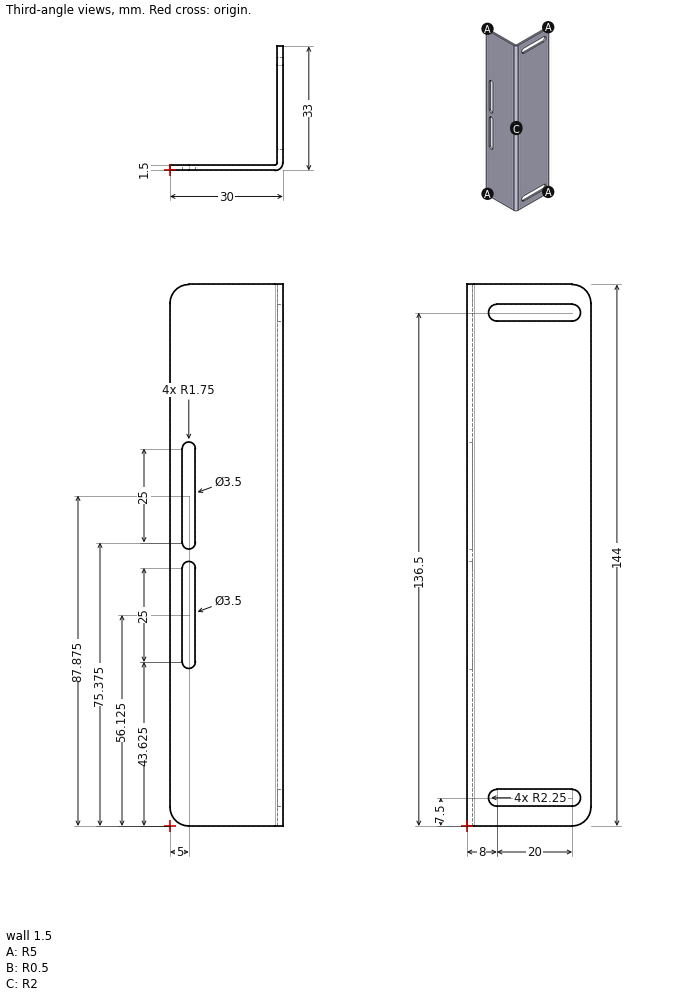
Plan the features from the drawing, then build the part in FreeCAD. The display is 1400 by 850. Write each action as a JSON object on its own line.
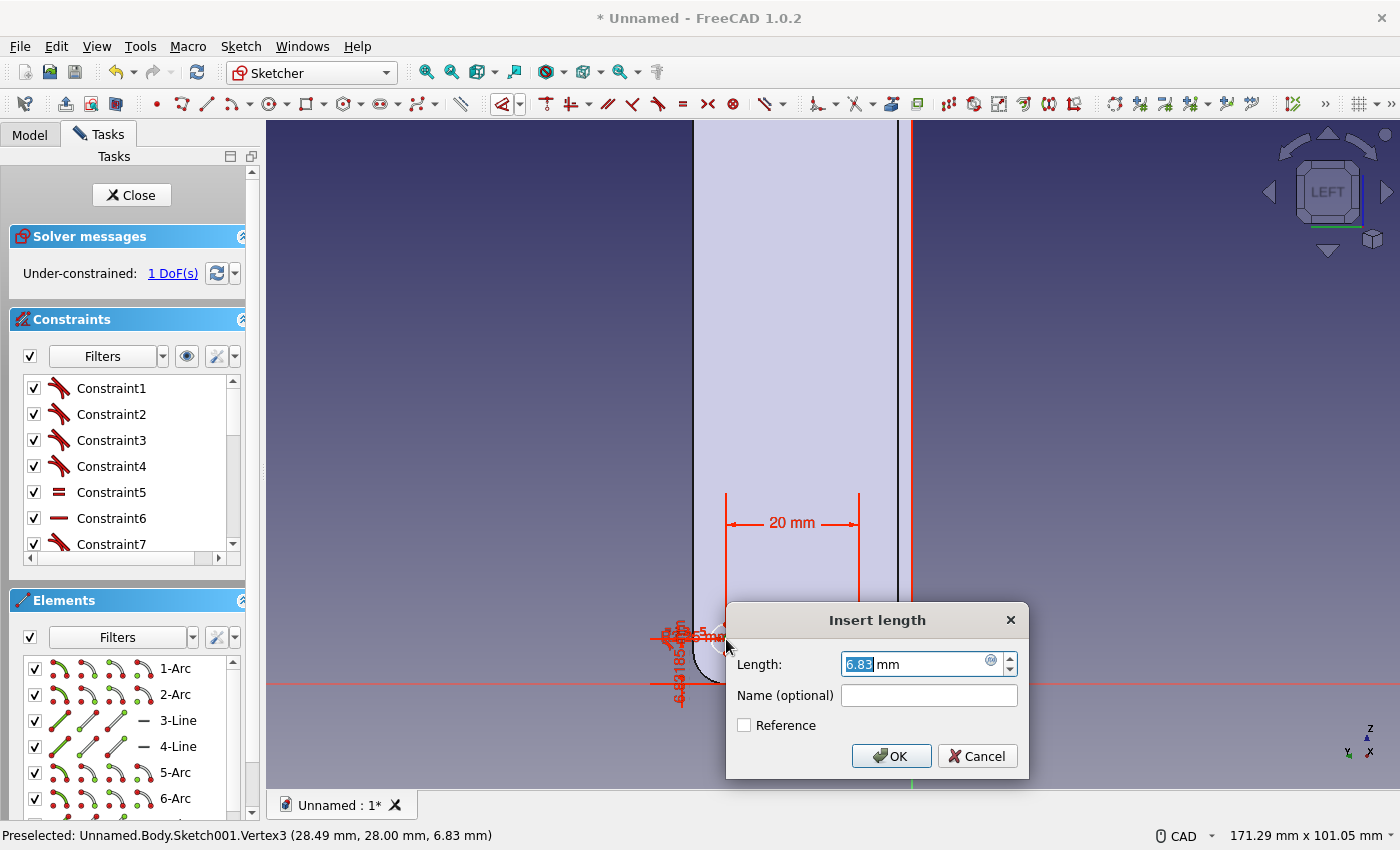
{"action": "type", "text": "7.5"}
{"action": "key", "text": "Return"}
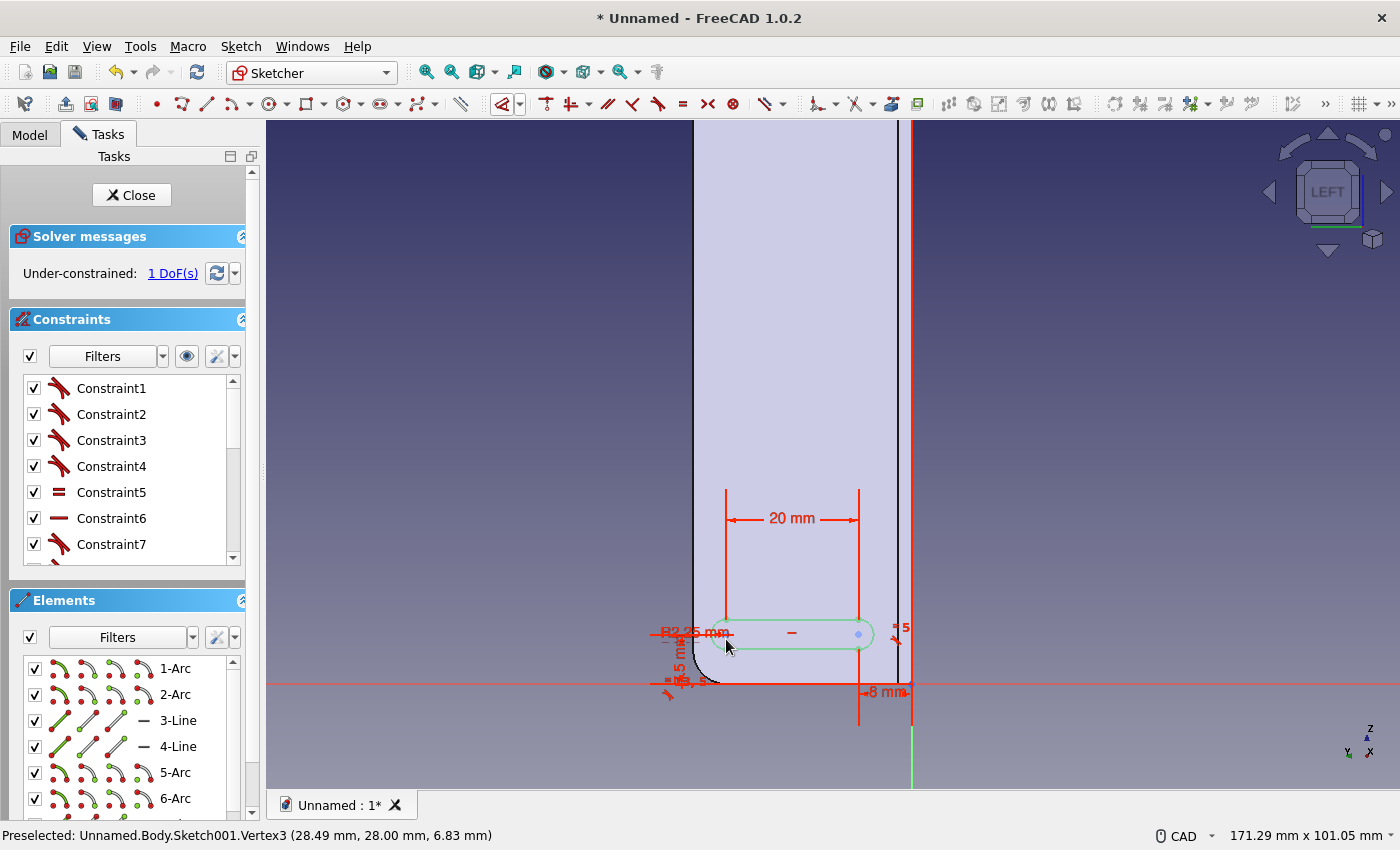
{"action": "scroll", "coordinate": [726, 642], "scroll_direction": "down", "scroll_amount": 4}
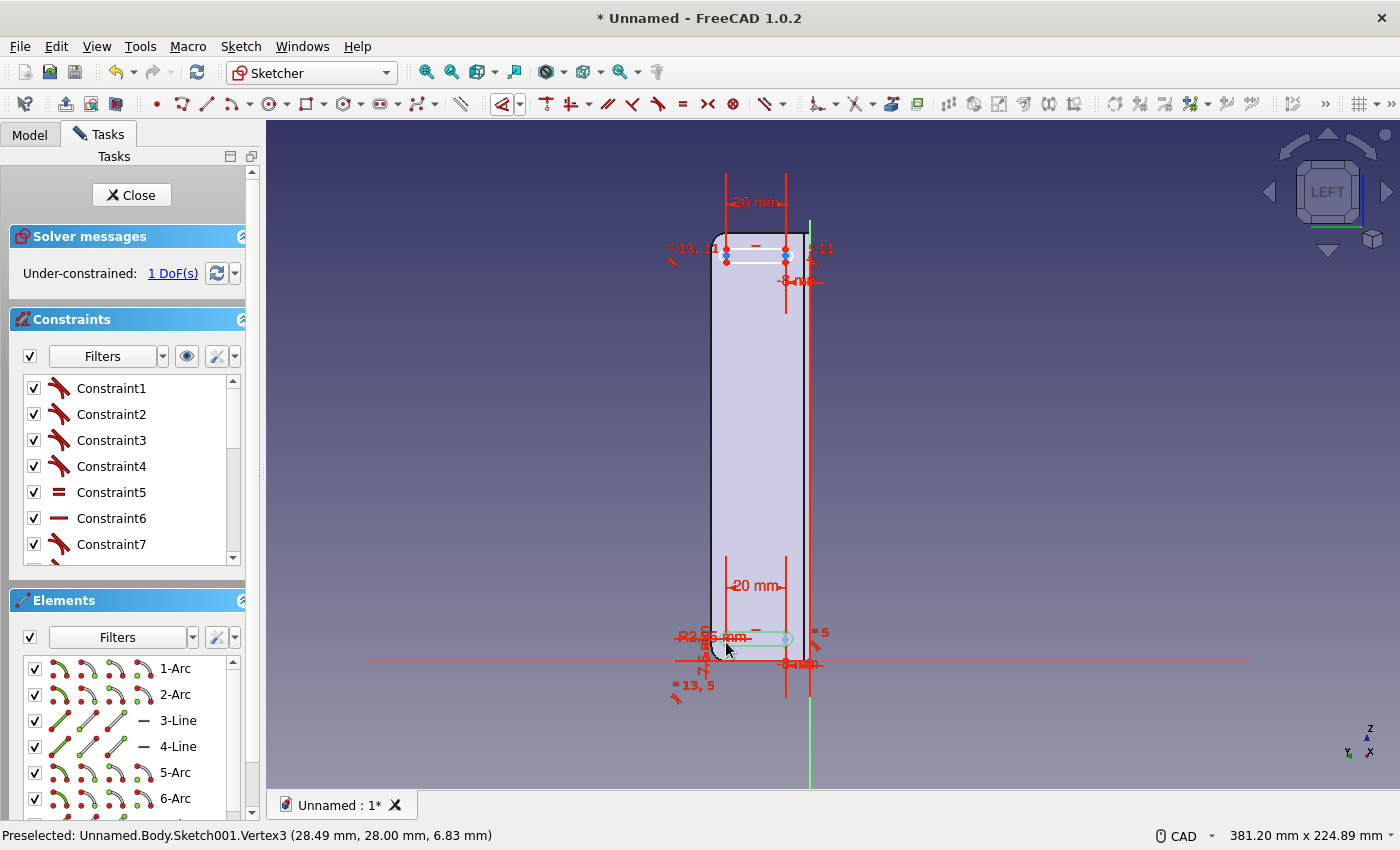
{"action": "scroll", "coordinate": [726, 256], "scroll_direction": "up", "scroll_amount": 4}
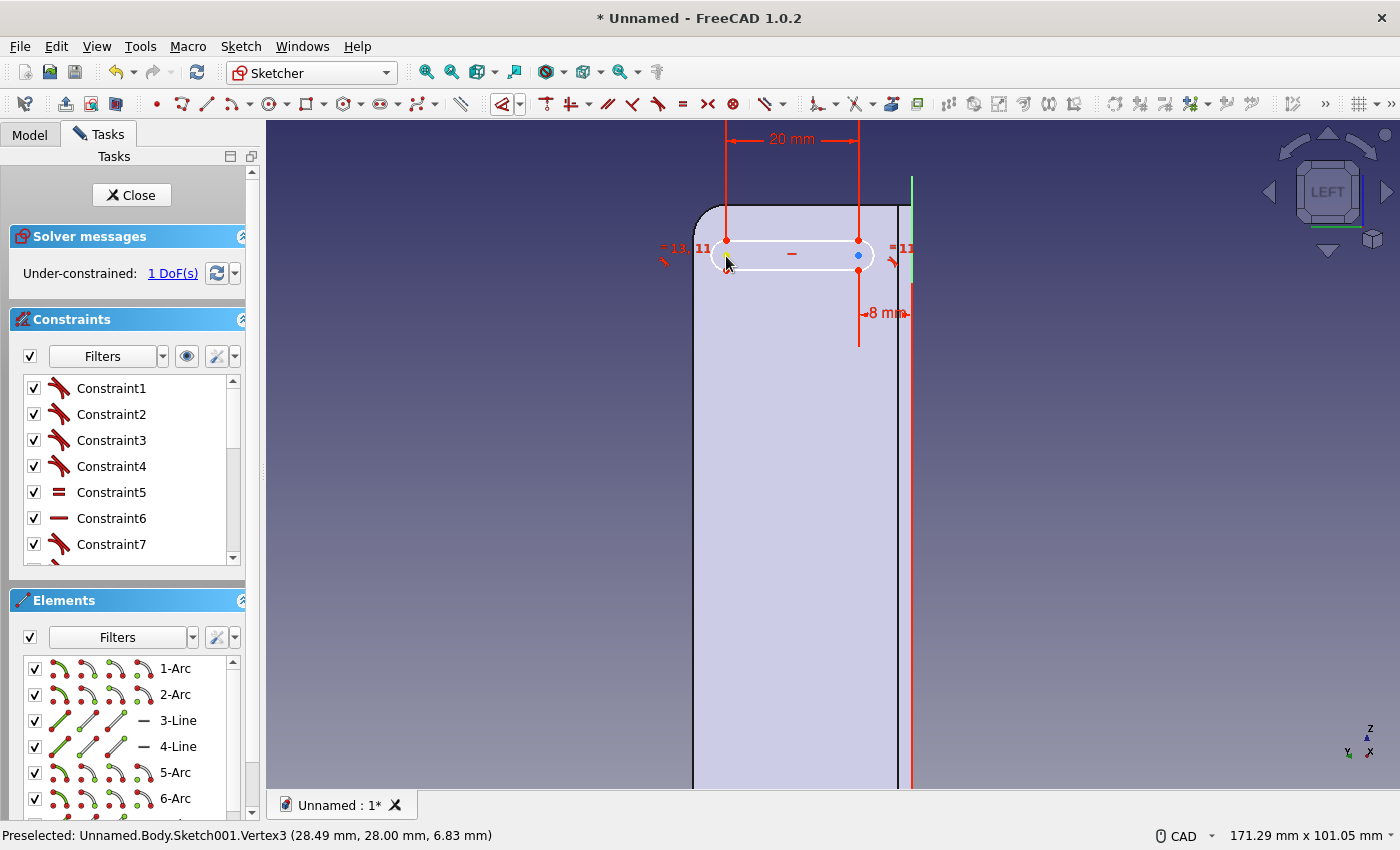
{"action": "left_click", "coordinate": [726, 255]}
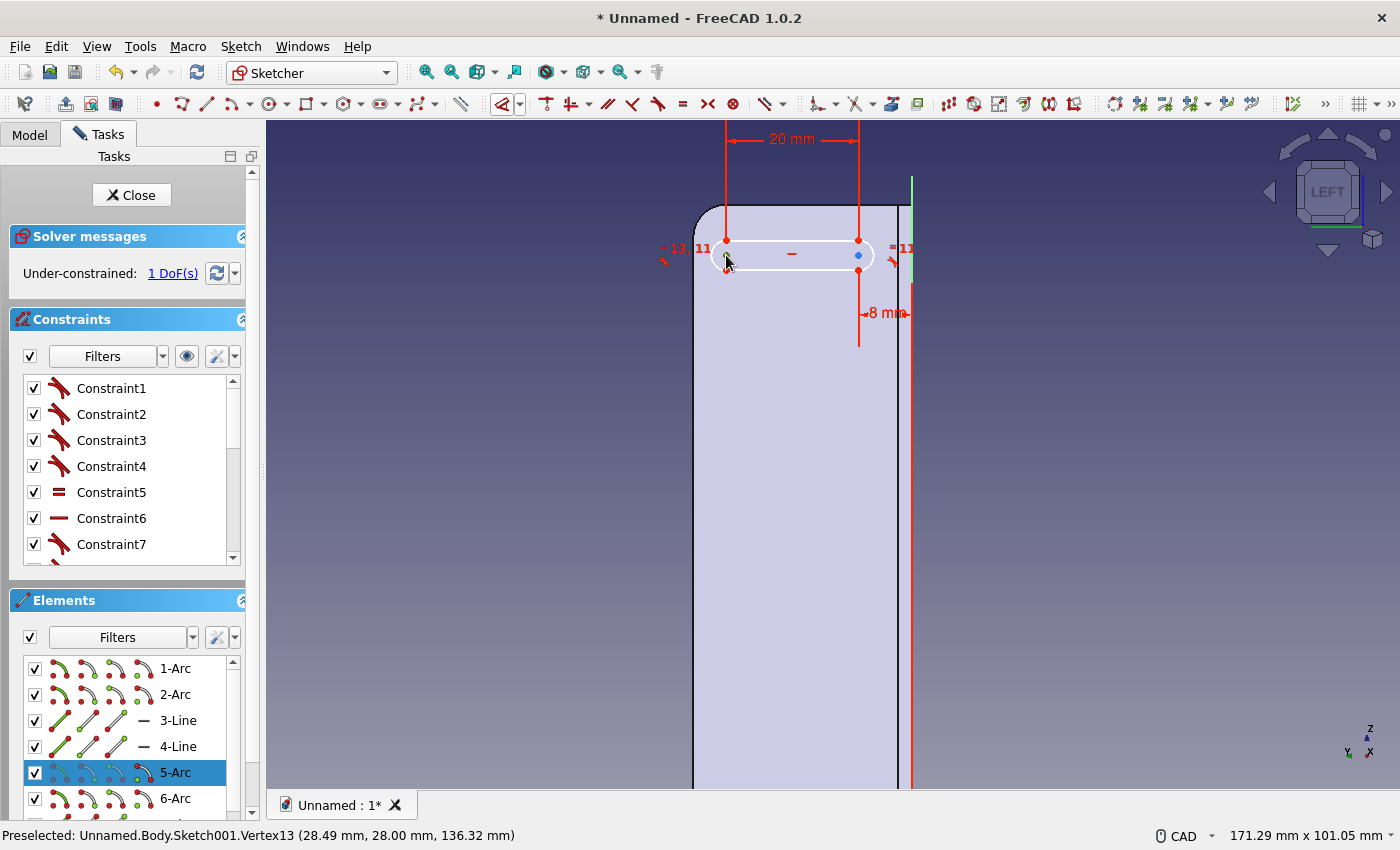
{"action": "key", "text": "i"}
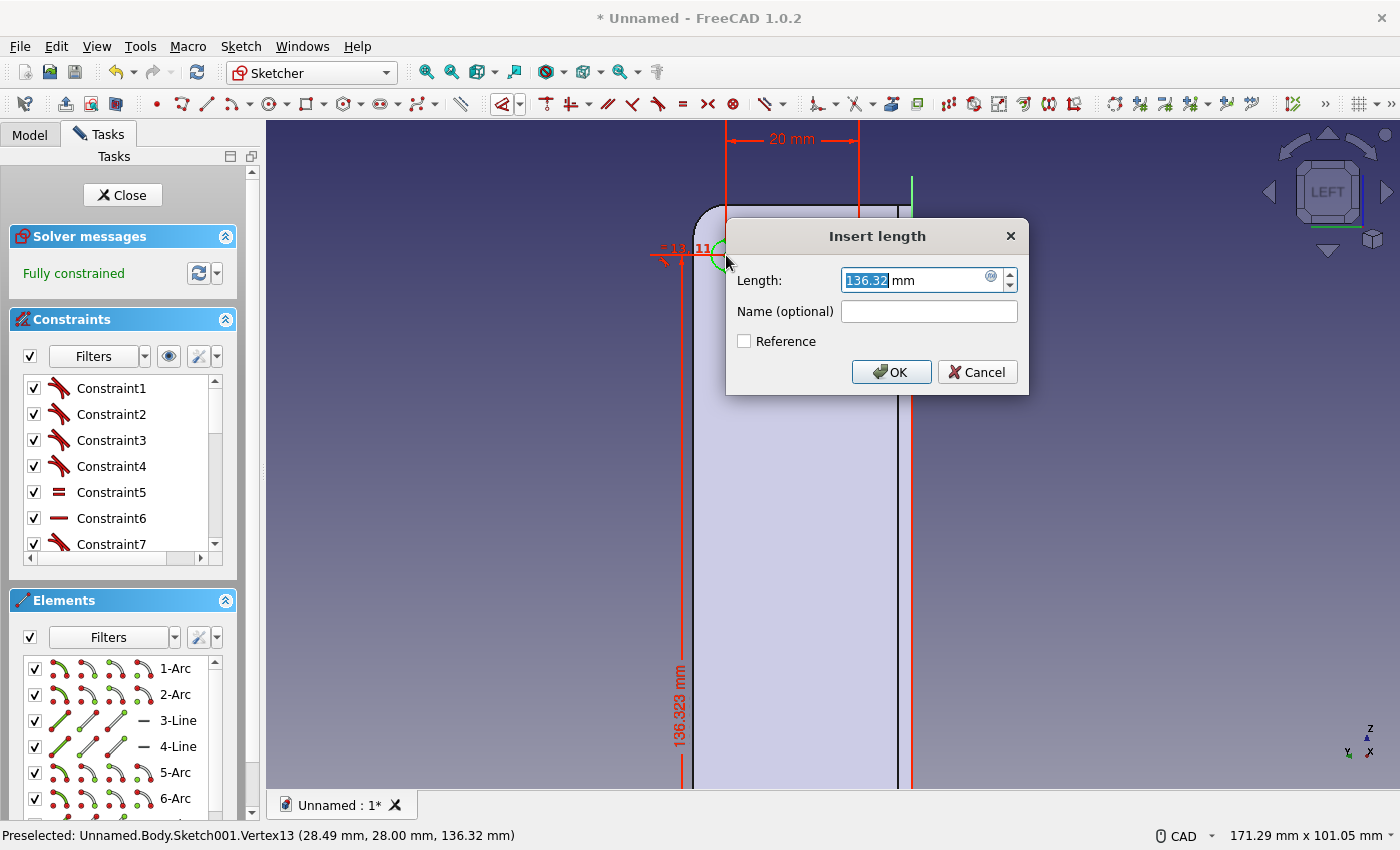
{"action": "type", "text": "136.5"}
{"action": "key", "text": "Return"}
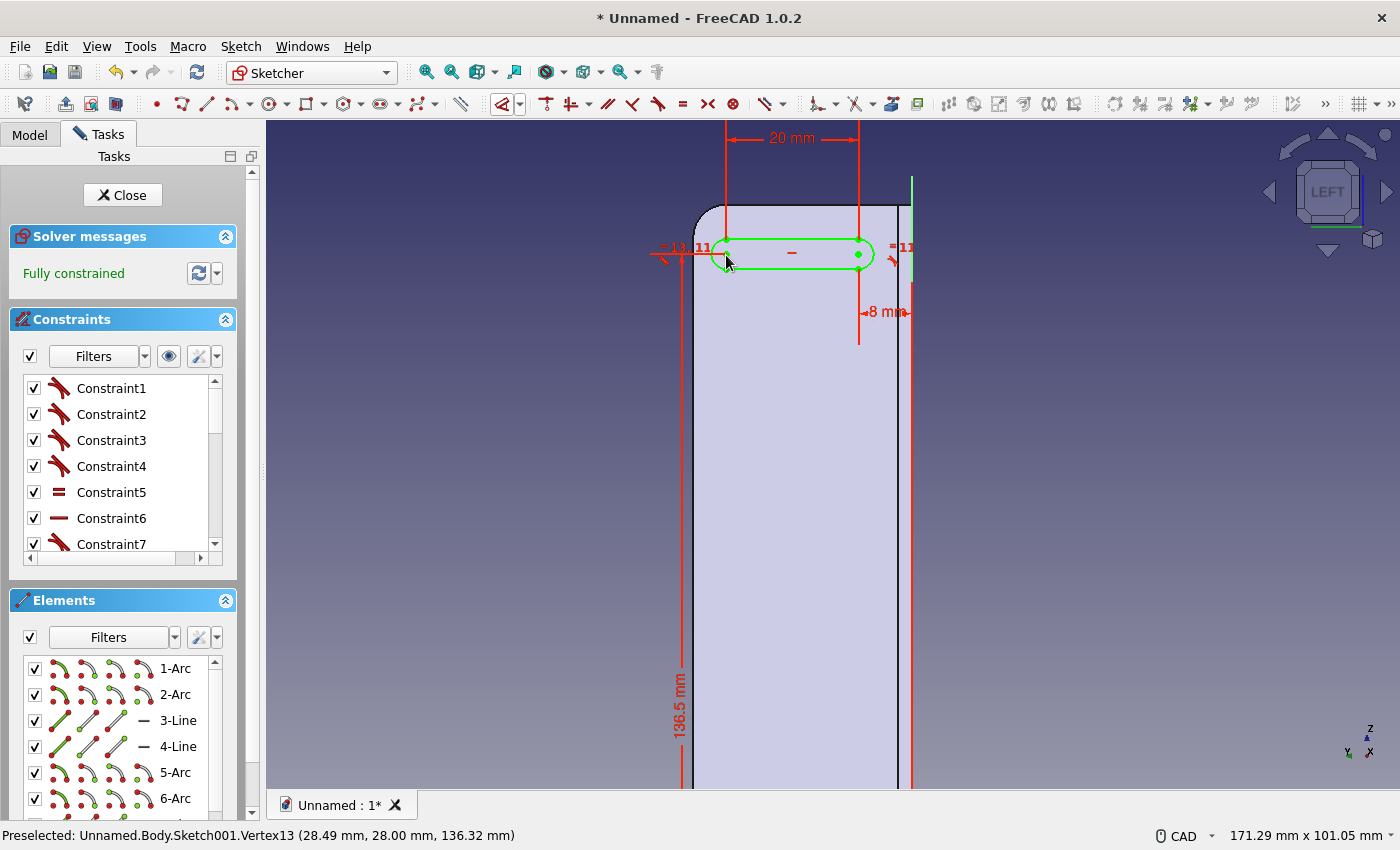
{"action": "left_click", "coordinate": [123, 195]}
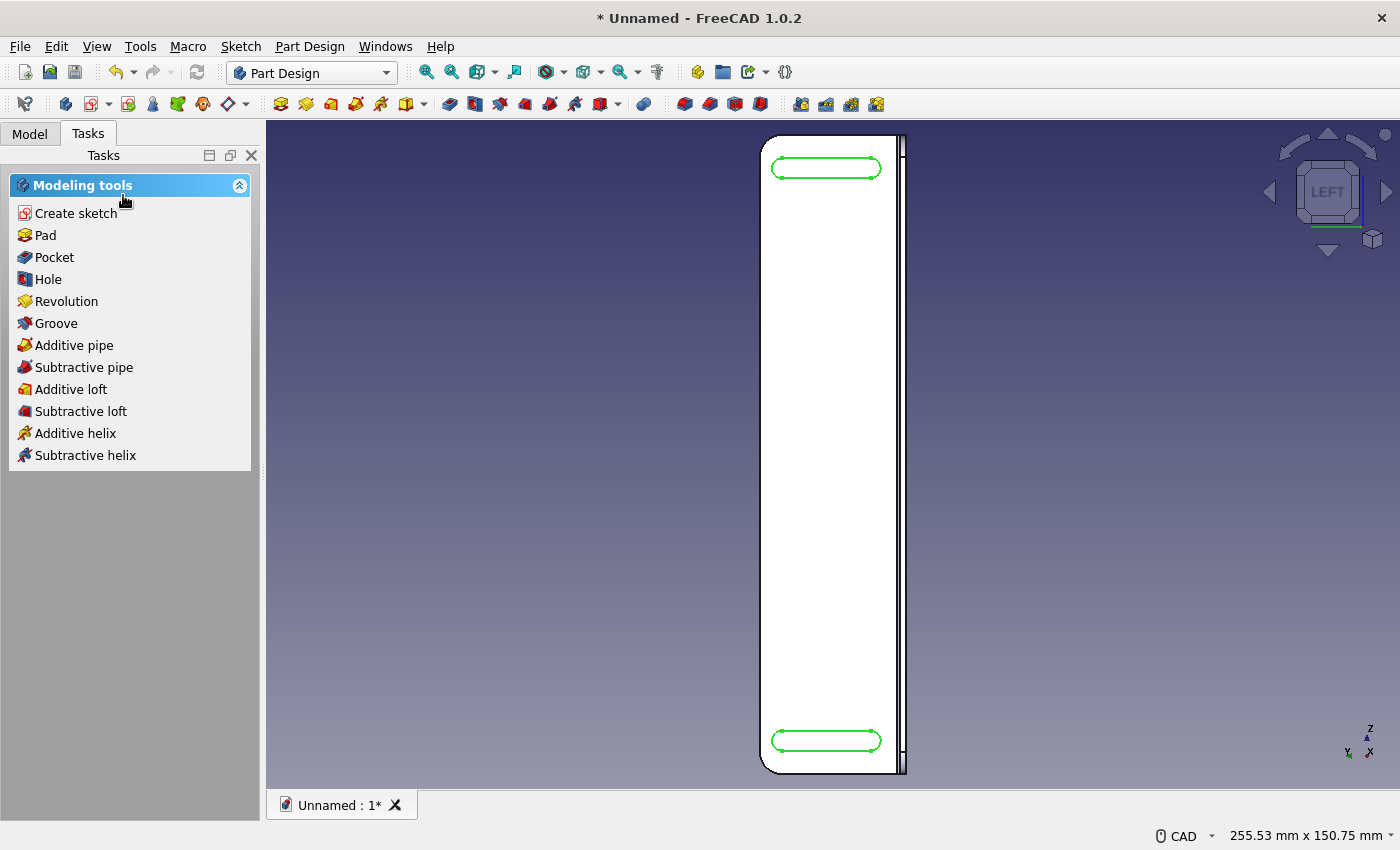
{"action": "left_click", "coordinate": [450, 104]}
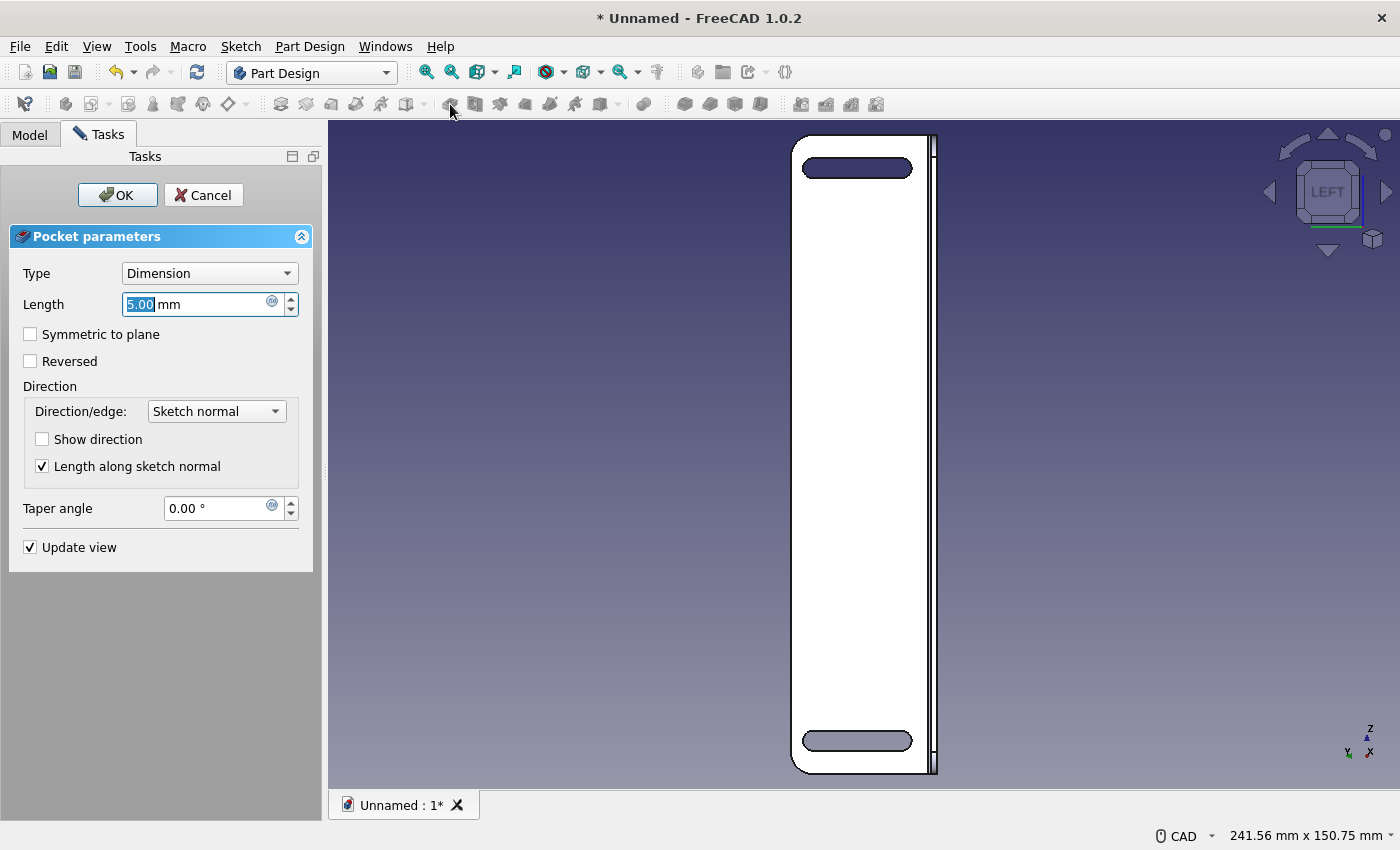
{"action": "left_click", "coordinate": [210, 274]}